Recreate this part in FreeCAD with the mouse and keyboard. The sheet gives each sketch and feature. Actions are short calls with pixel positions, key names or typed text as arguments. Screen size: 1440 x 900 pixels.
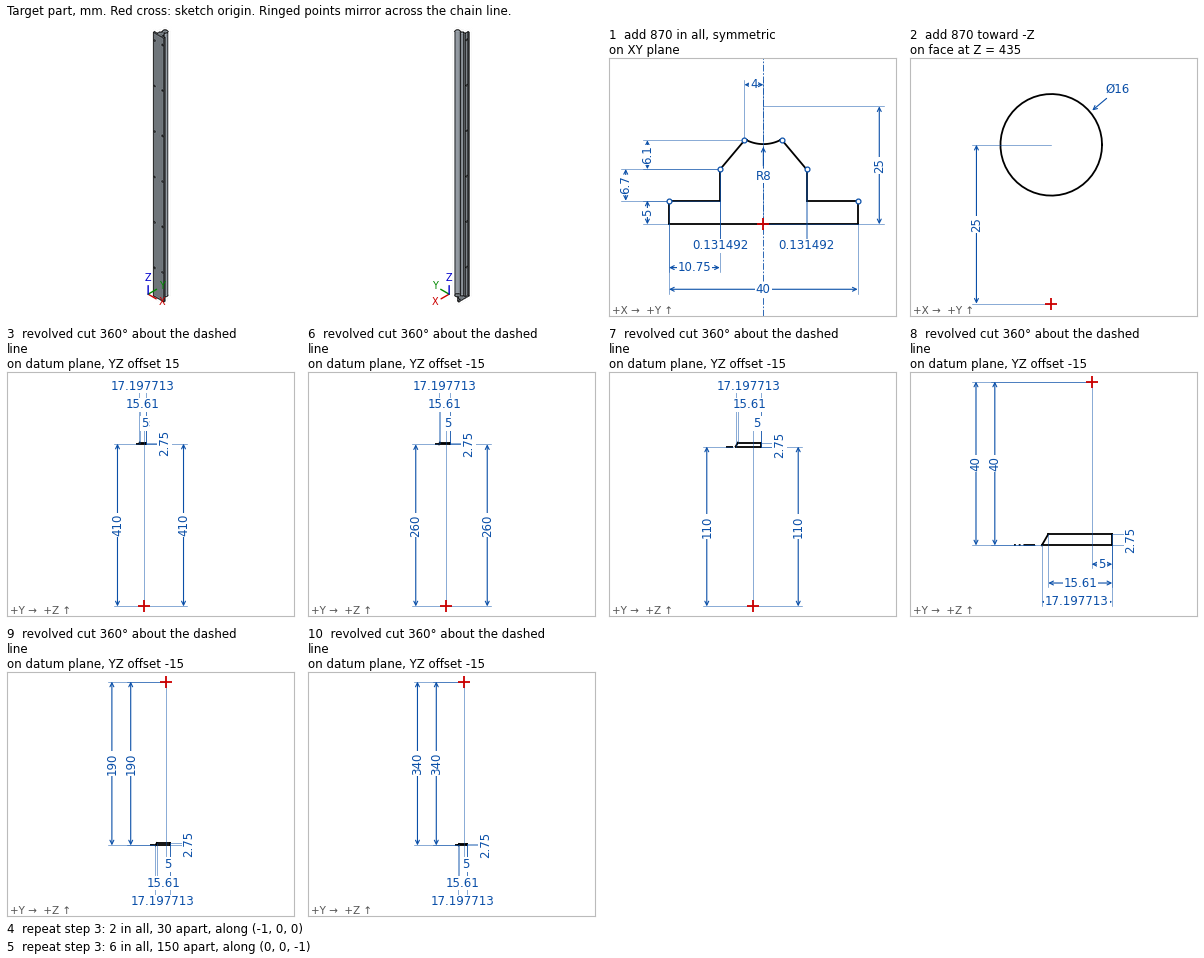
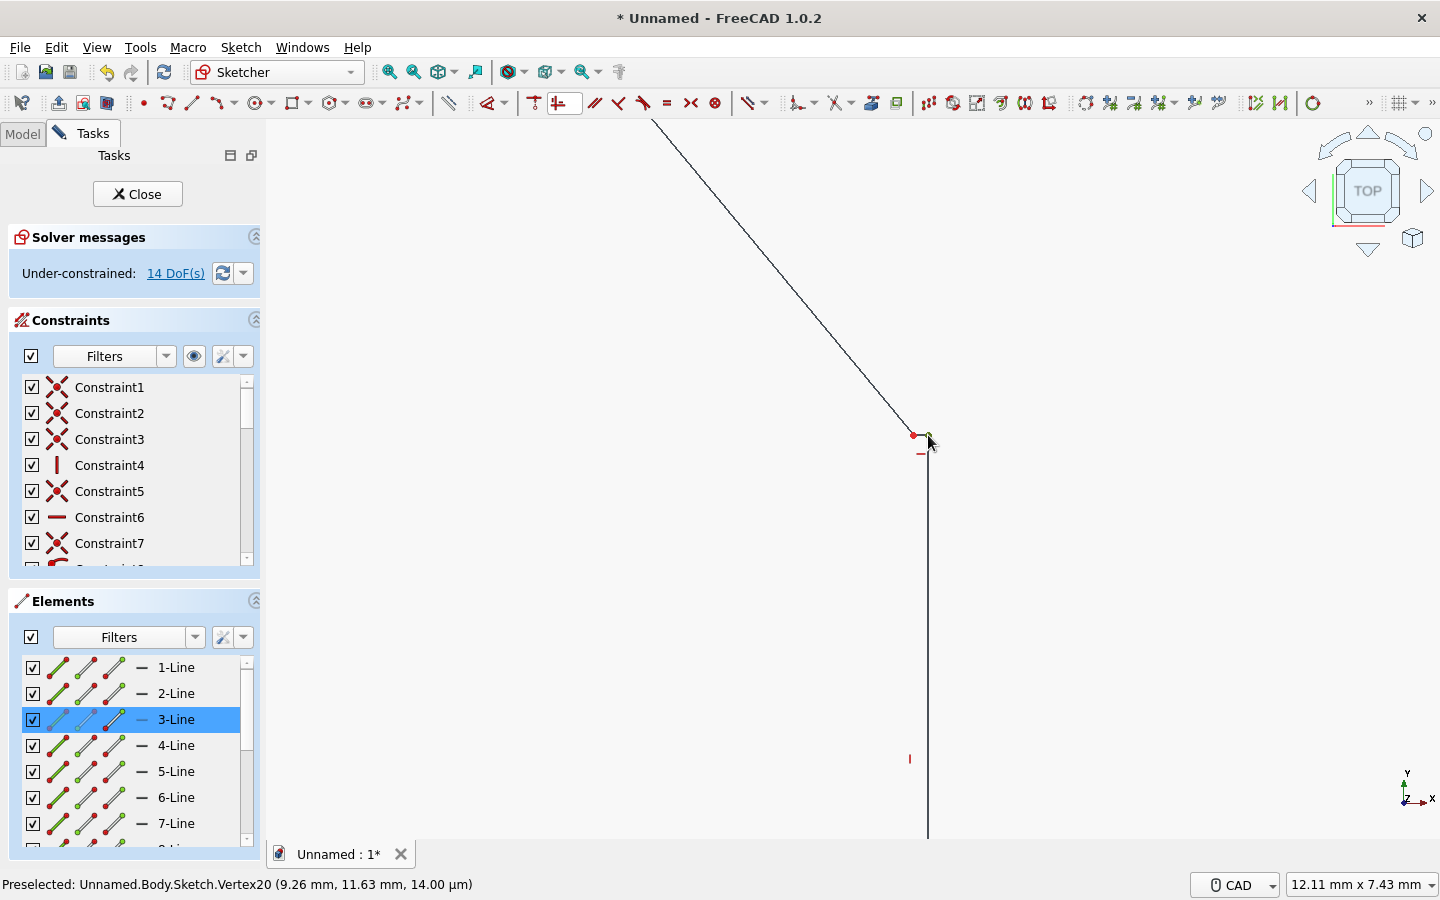
scroll(934, 435, down, 9)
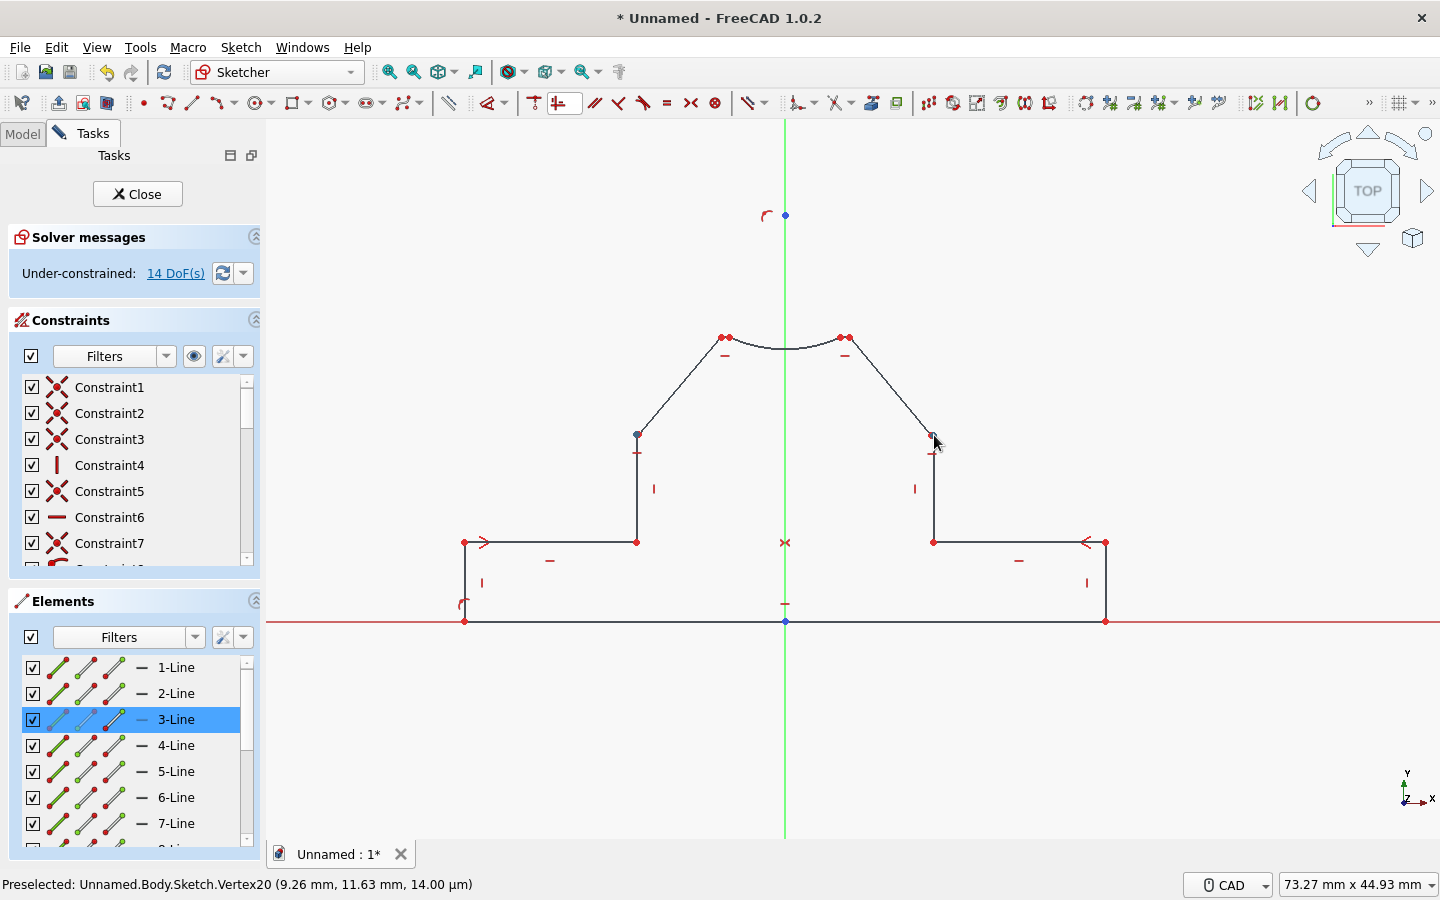
click(785, 764)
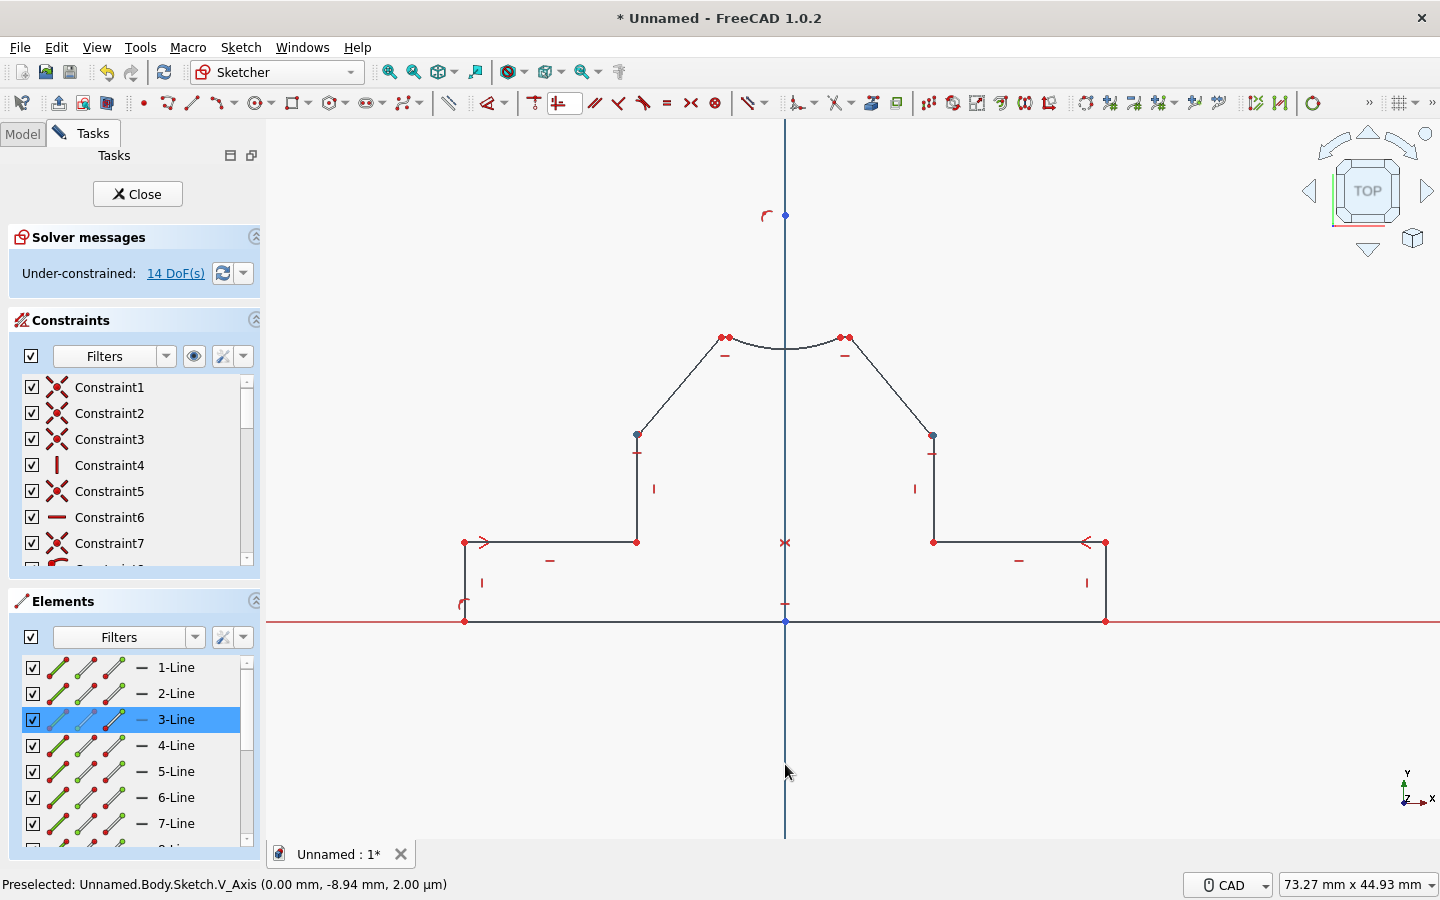
key(s)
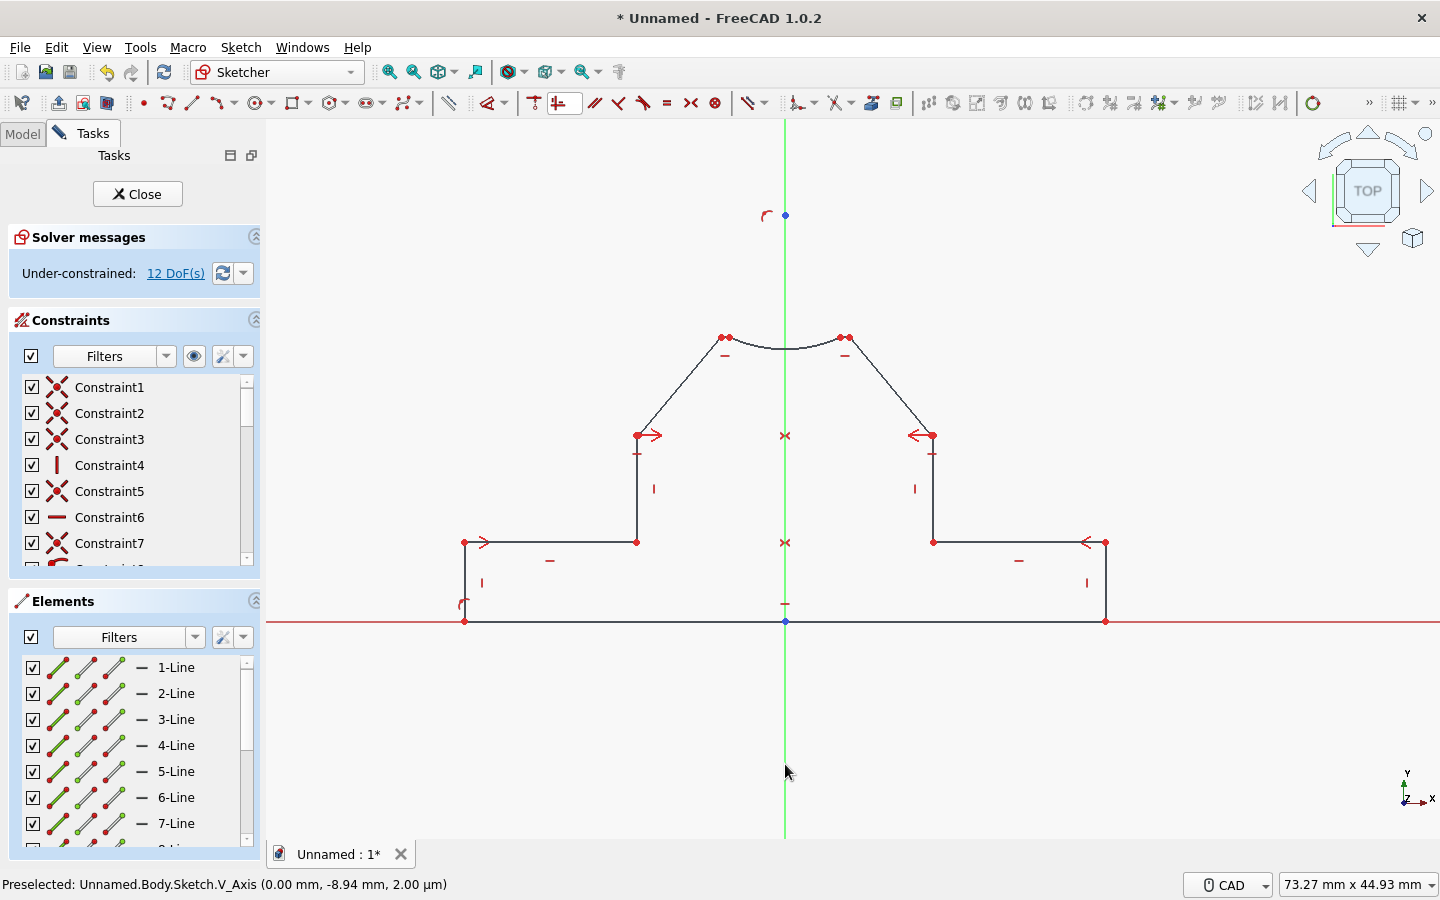
scroll(721, 337, up, 2)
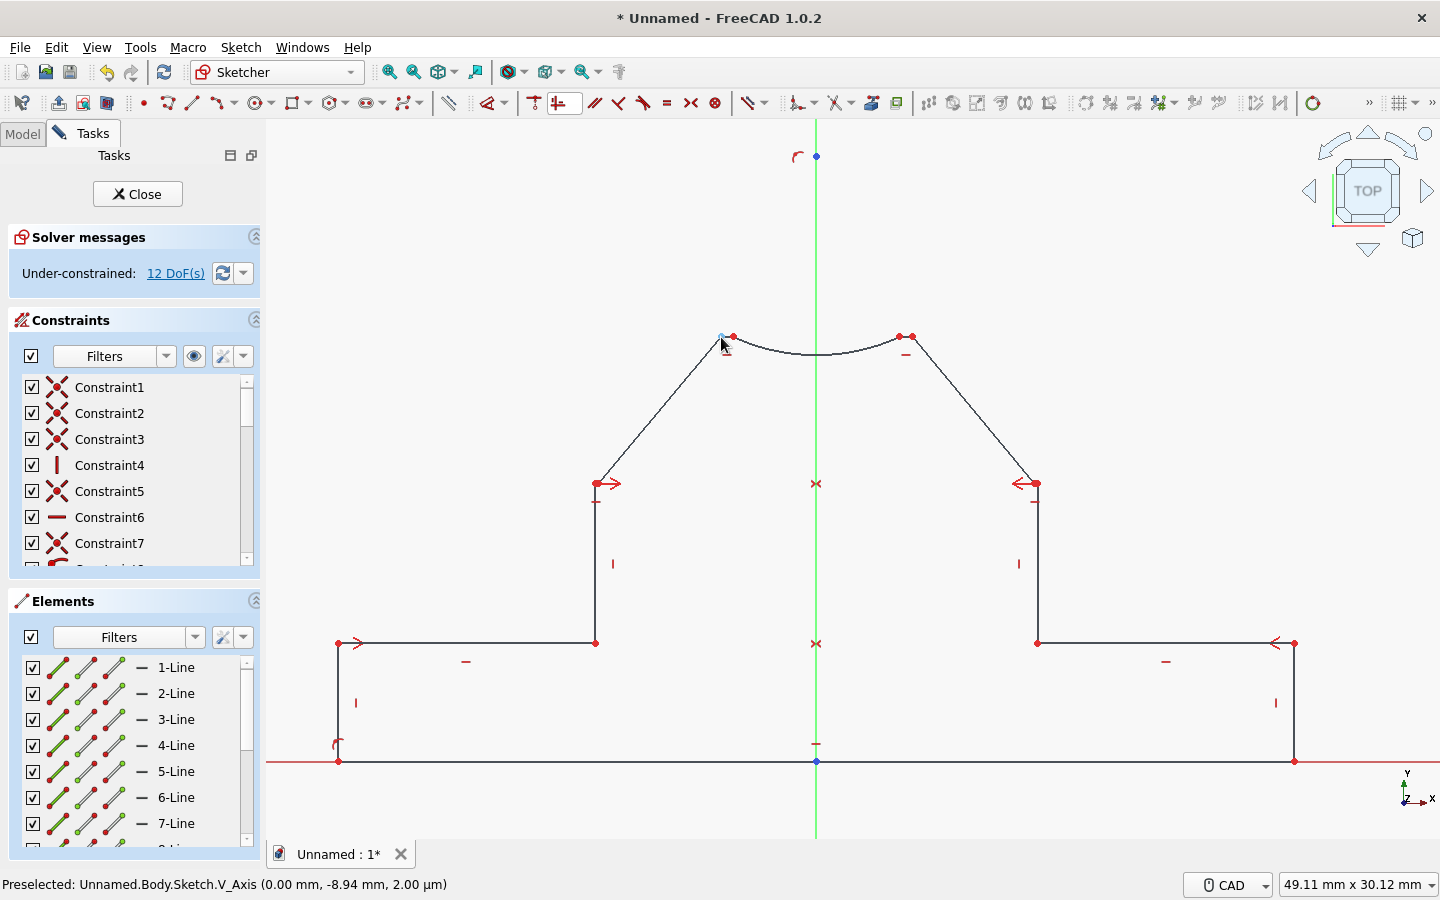
click(721, 337)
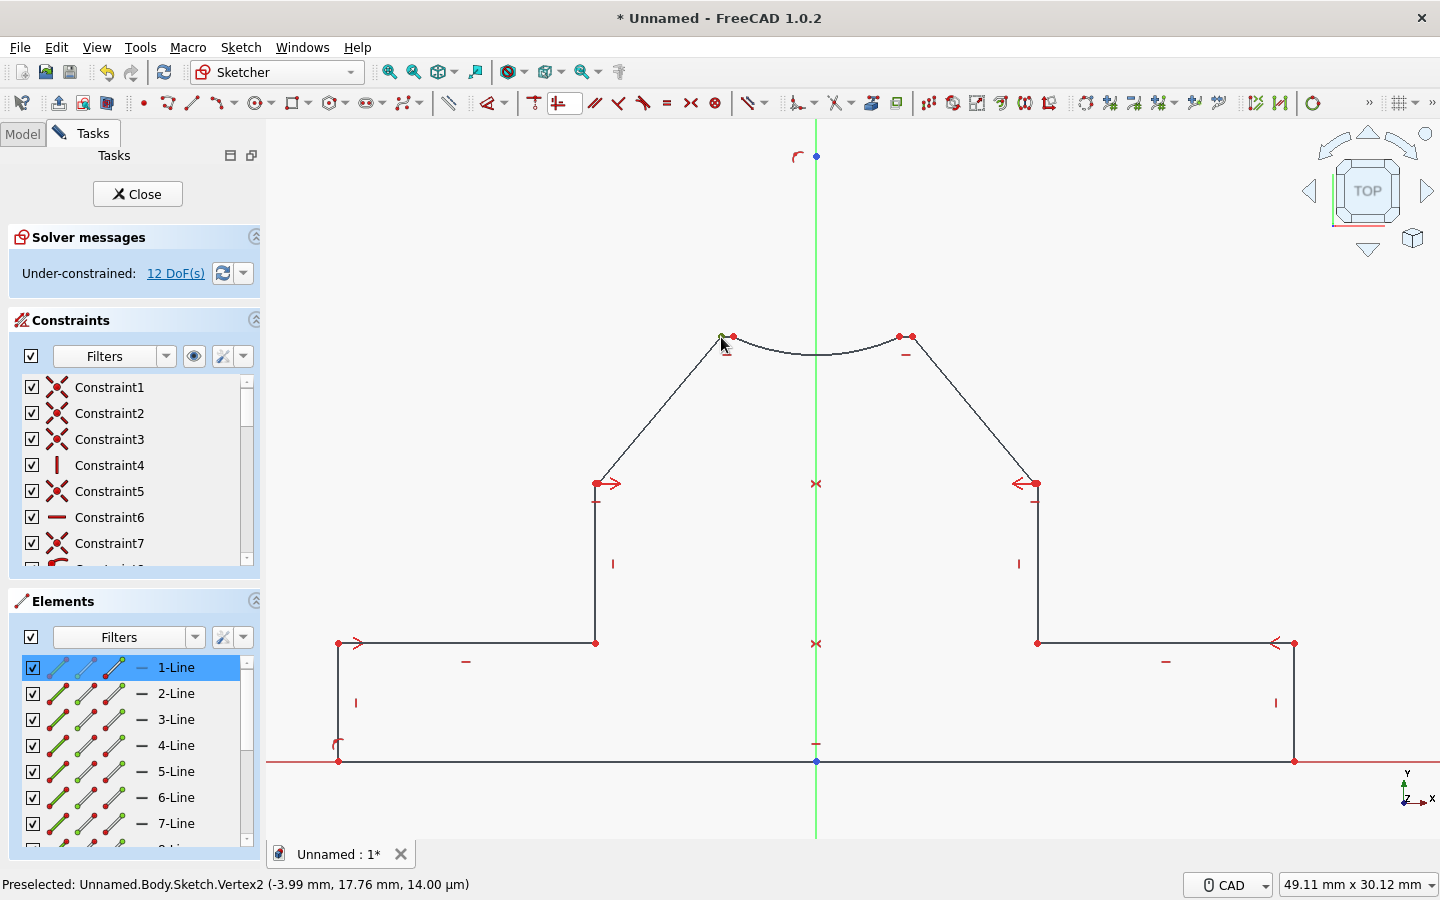
click(913, 337)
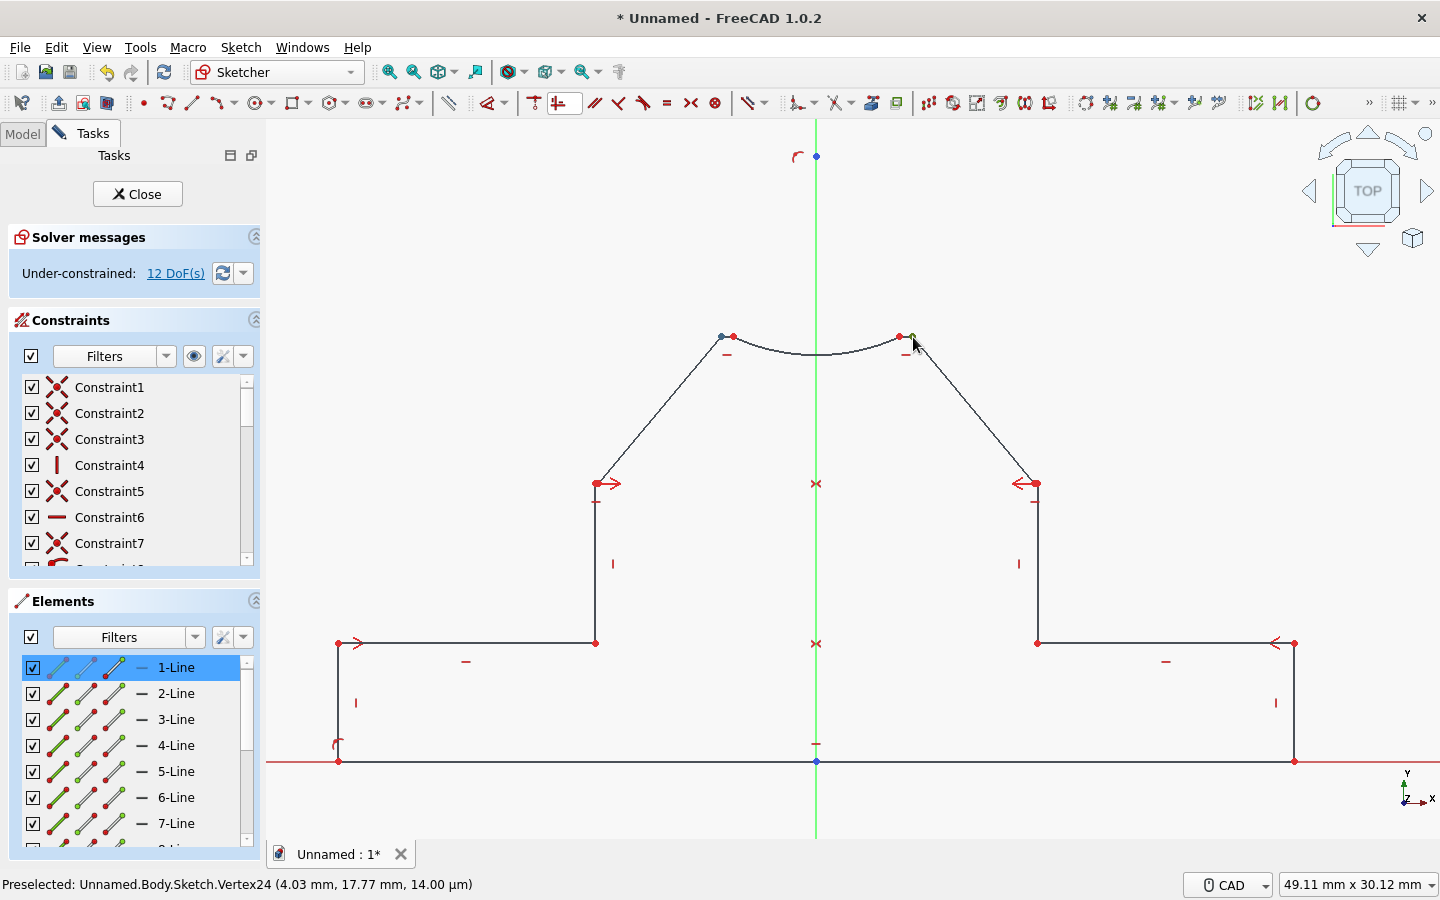
click(816, 716)